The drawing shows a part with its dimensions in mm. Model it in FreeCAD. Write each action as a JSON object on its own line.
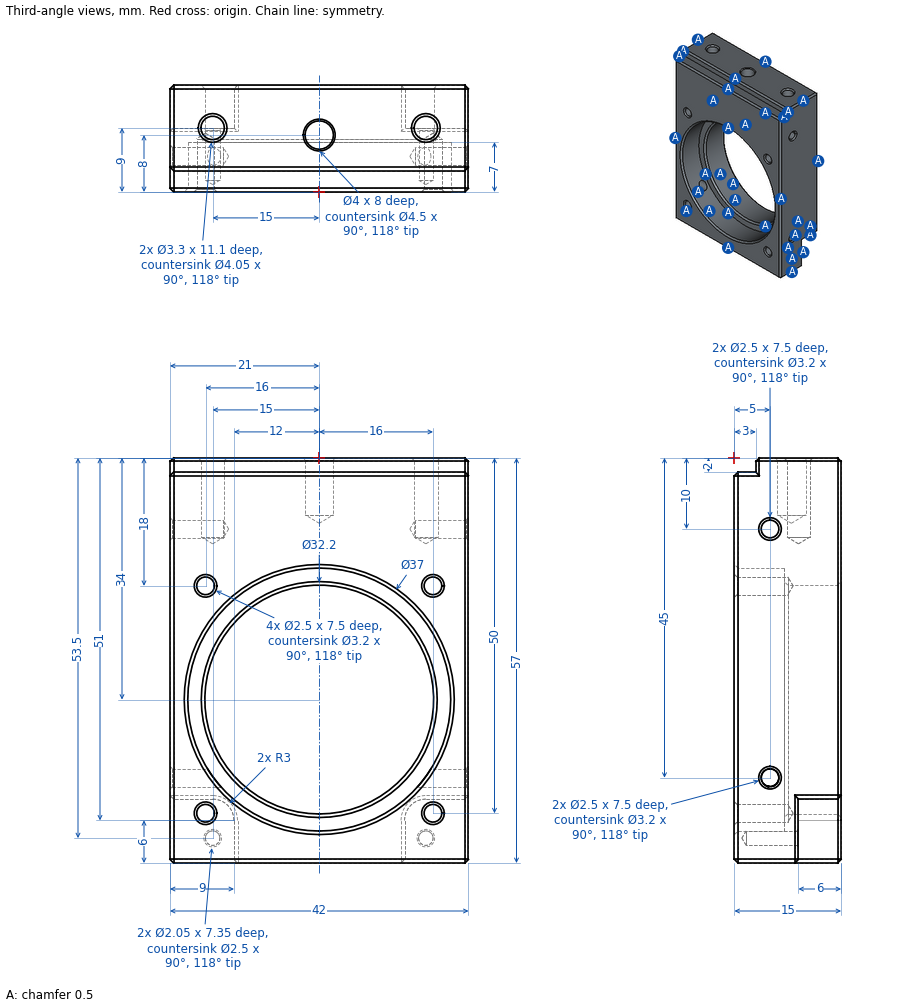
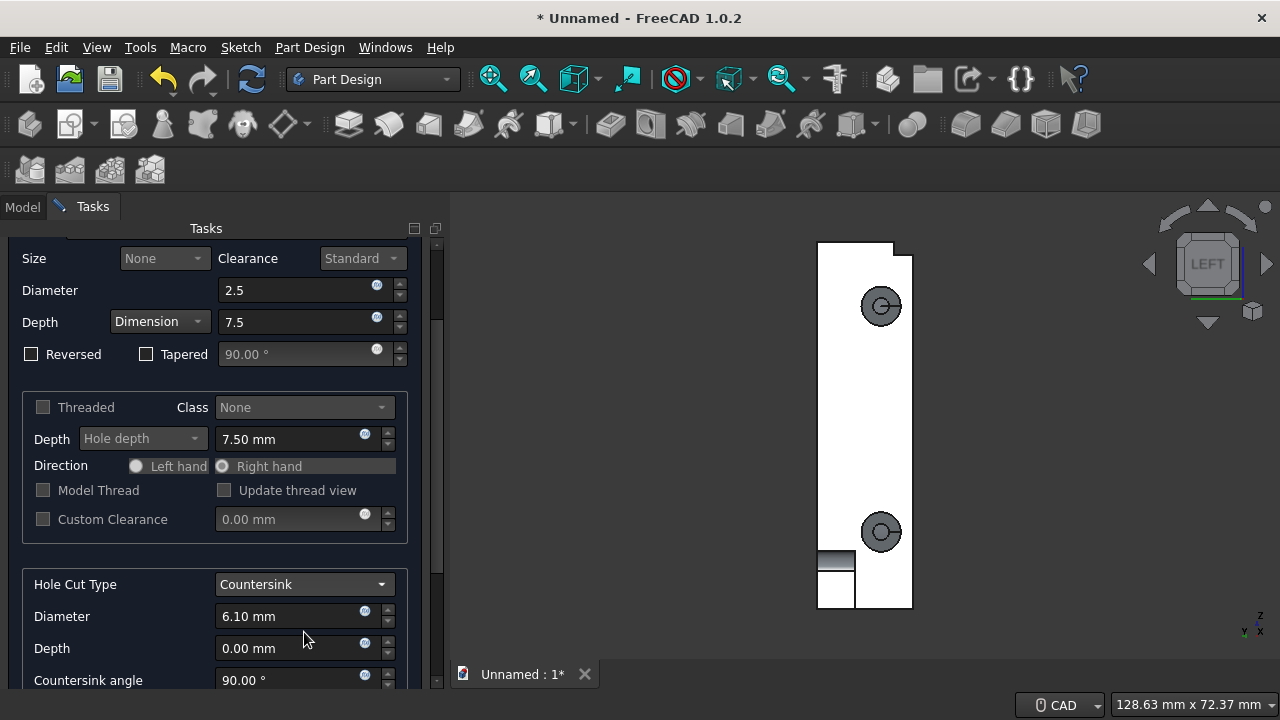
{"action": "triple_click", "coordinate": [298, 616]}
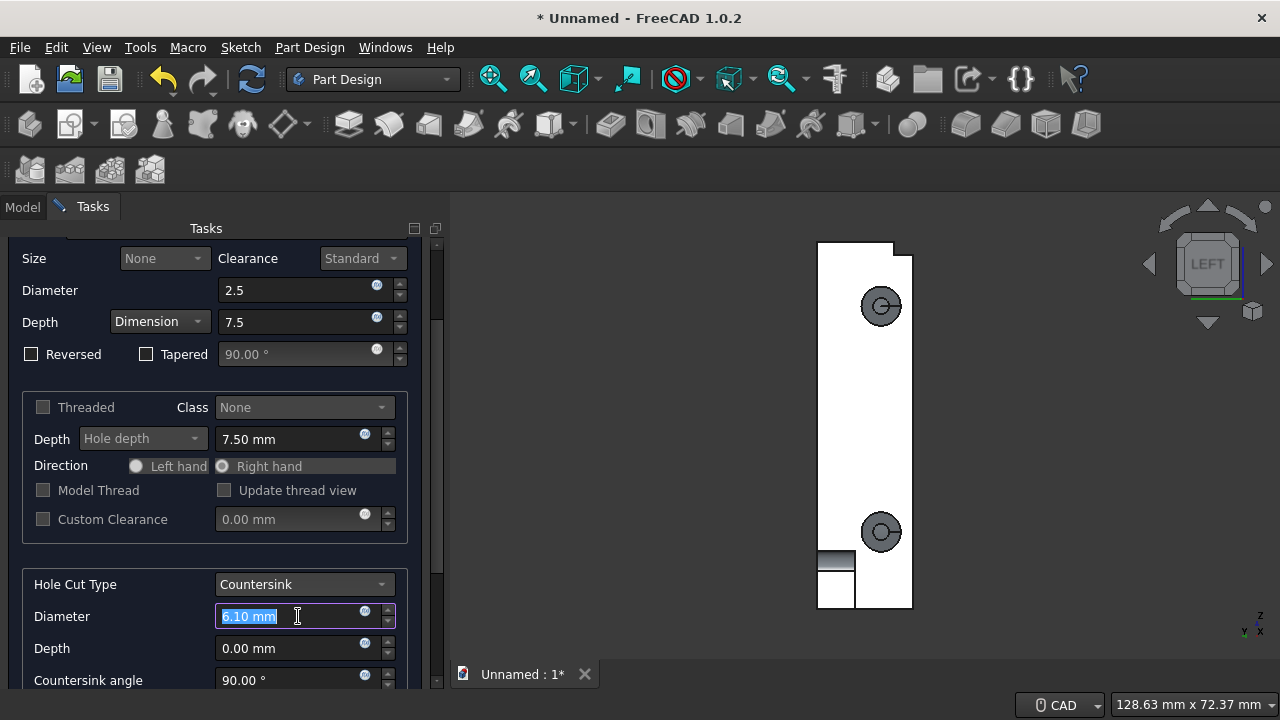
{"action": "type", "text": "3.2"}
{"action": "key", "text": "Tab"}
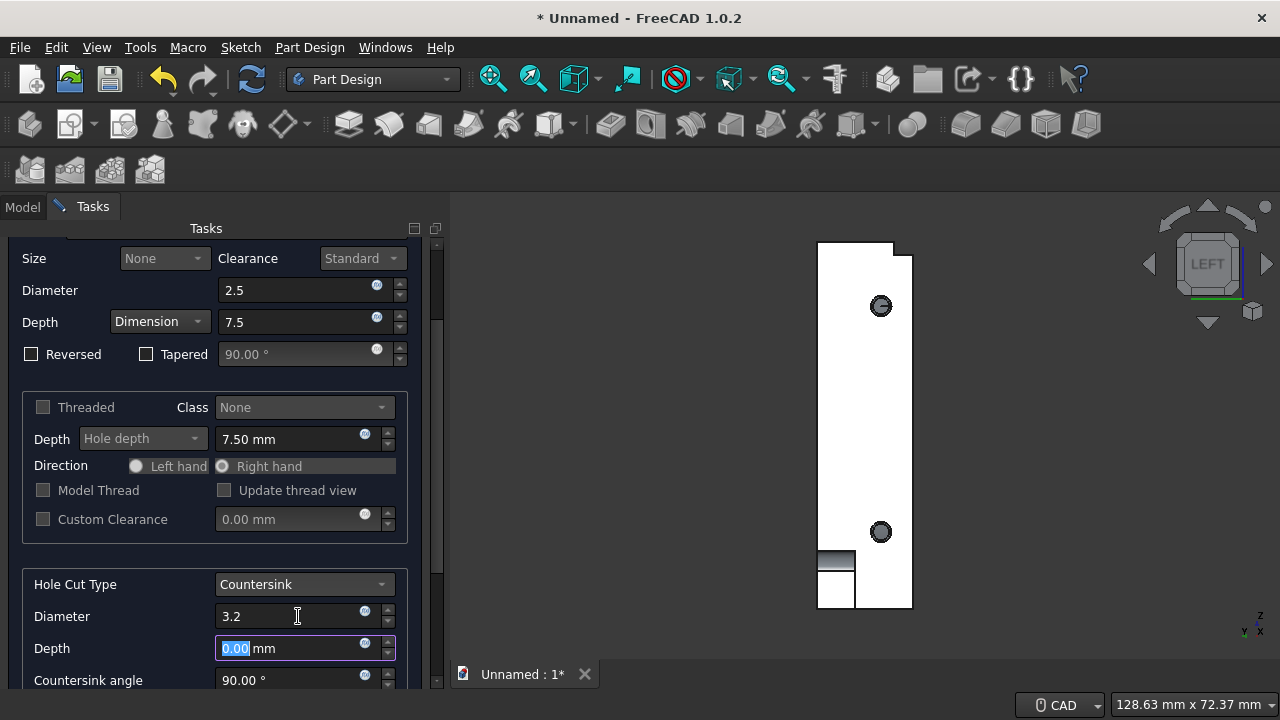
{"action": "scroll", "coordinate": [437, 463], "scroll_direction": "up", "scroll_amount": 3}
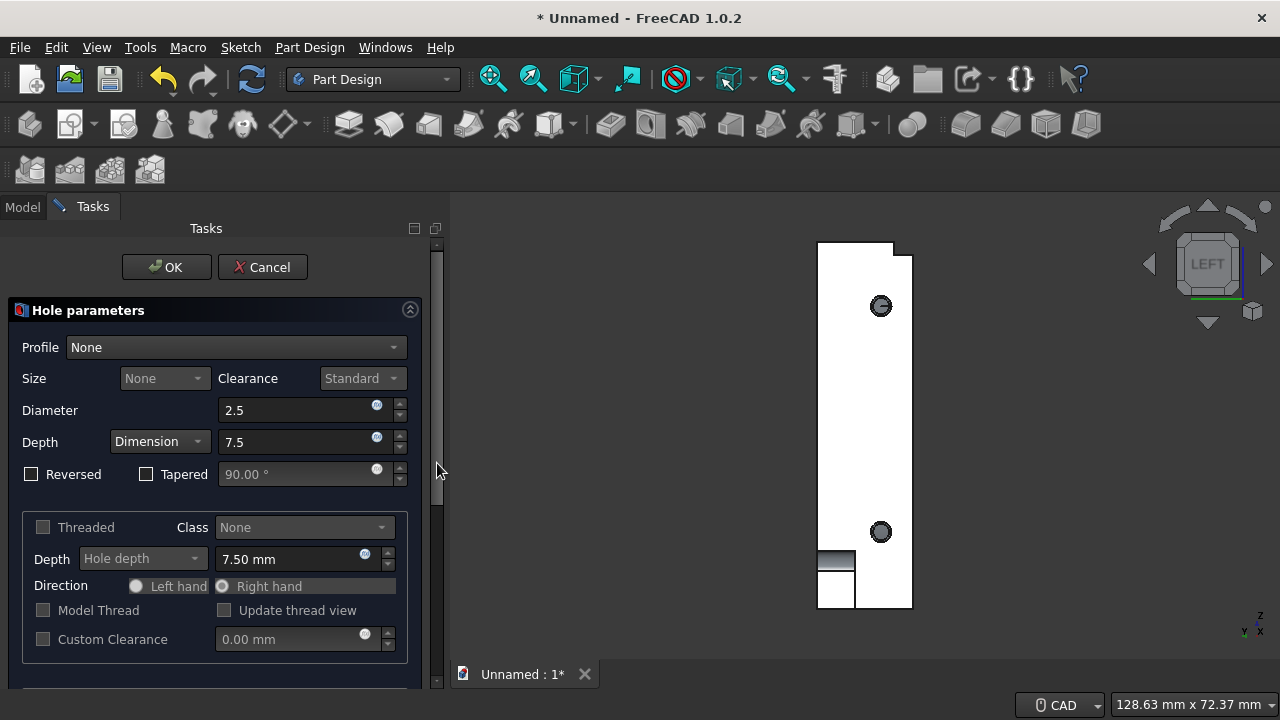
{"action": "left_click", "coordinate": [167, 267]}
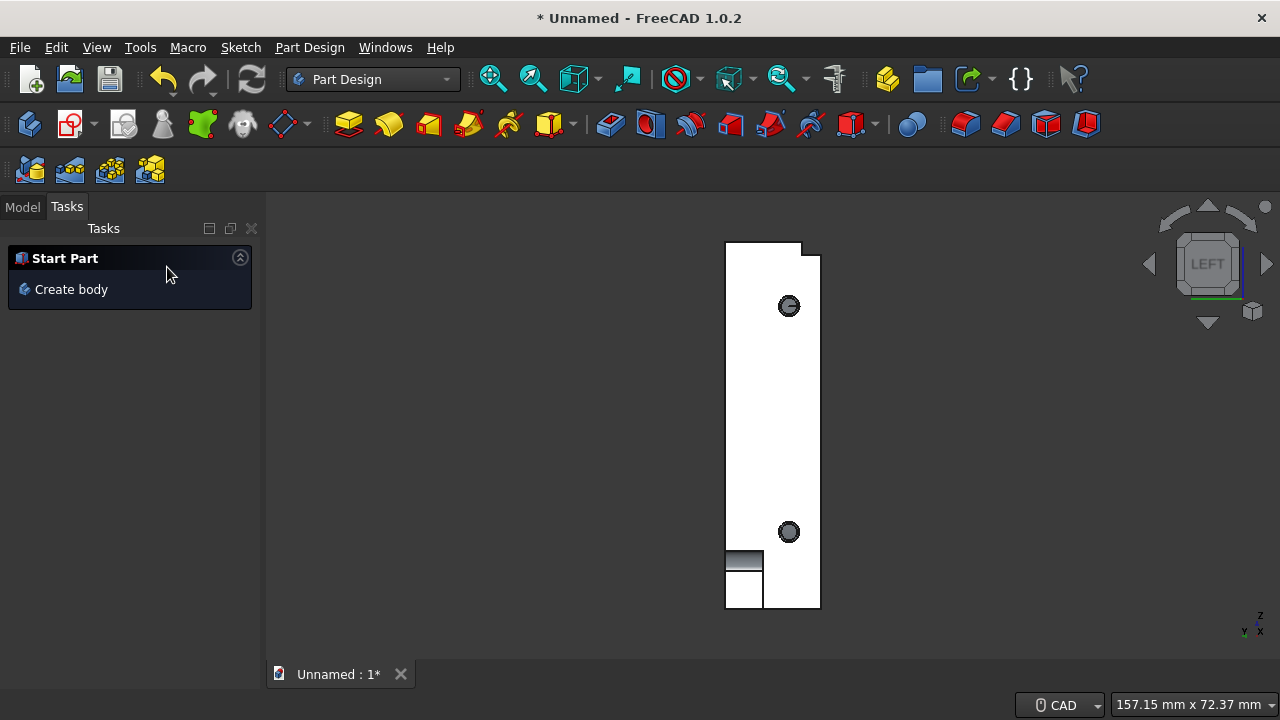
{"action": "key", "text": "0"}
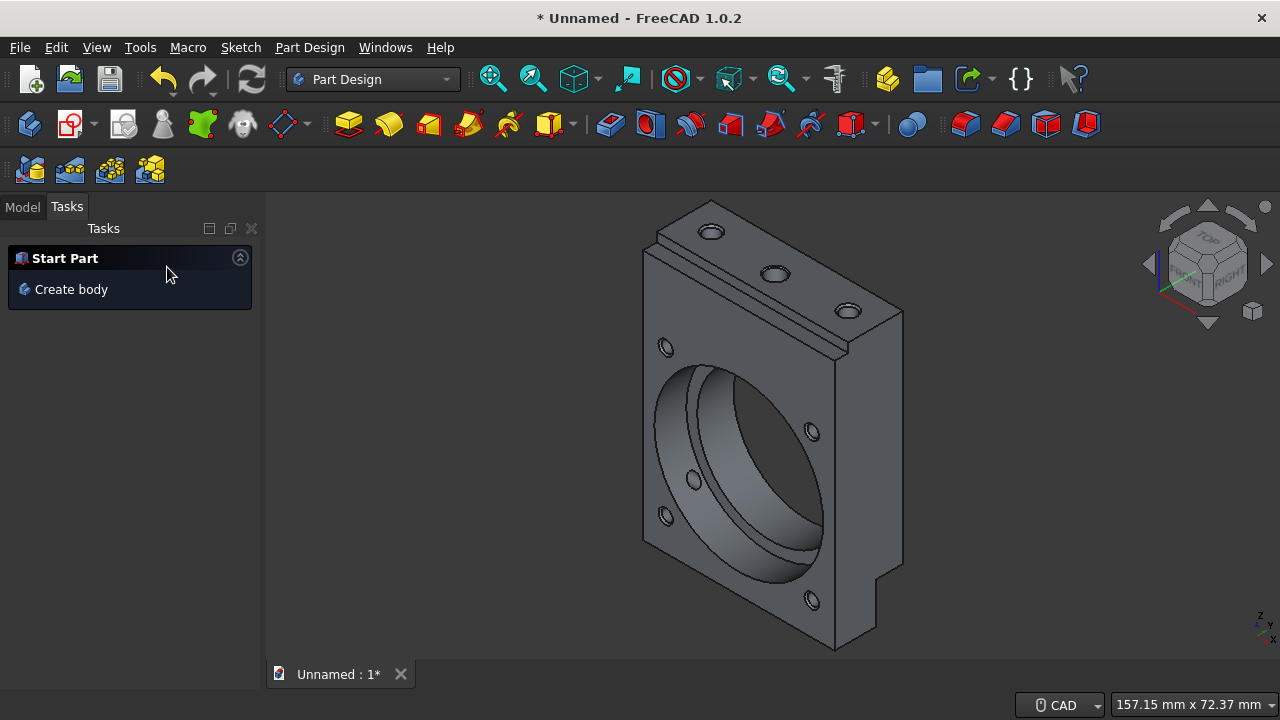
{"action": "left_click", "coordinate": [869, 394]}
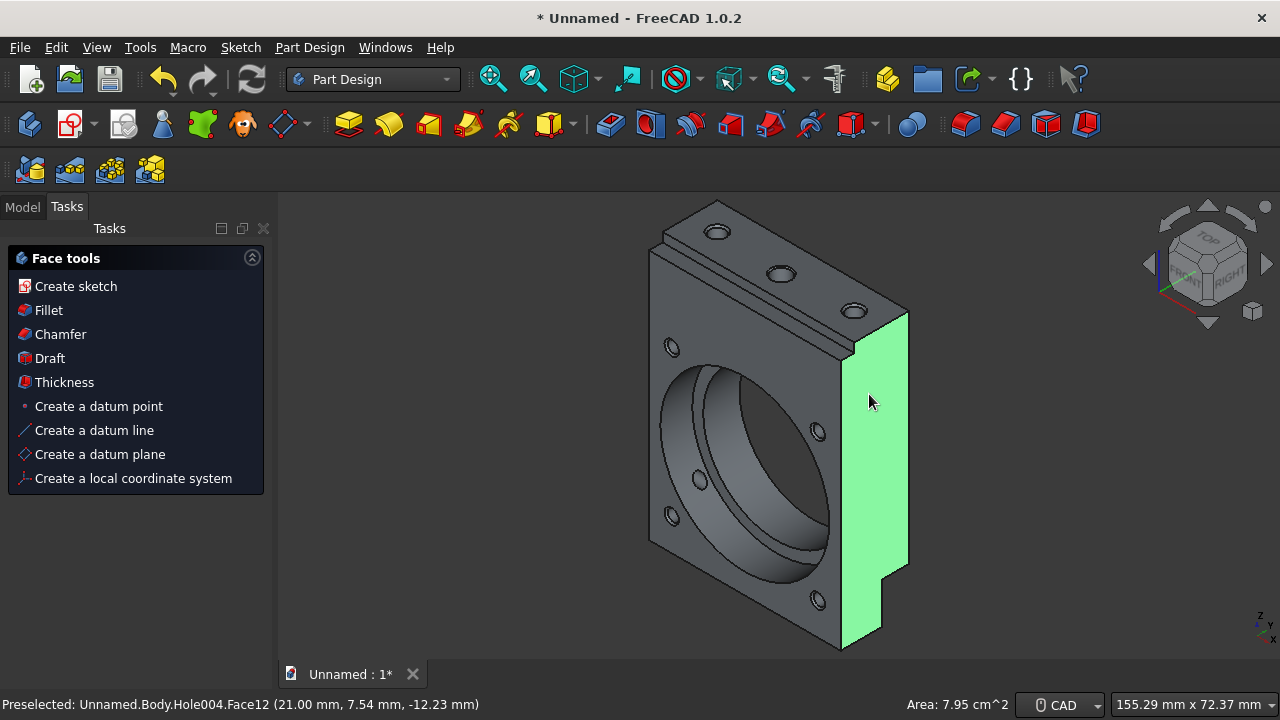
{"action": "left_click", "coordinate": [70, 124]}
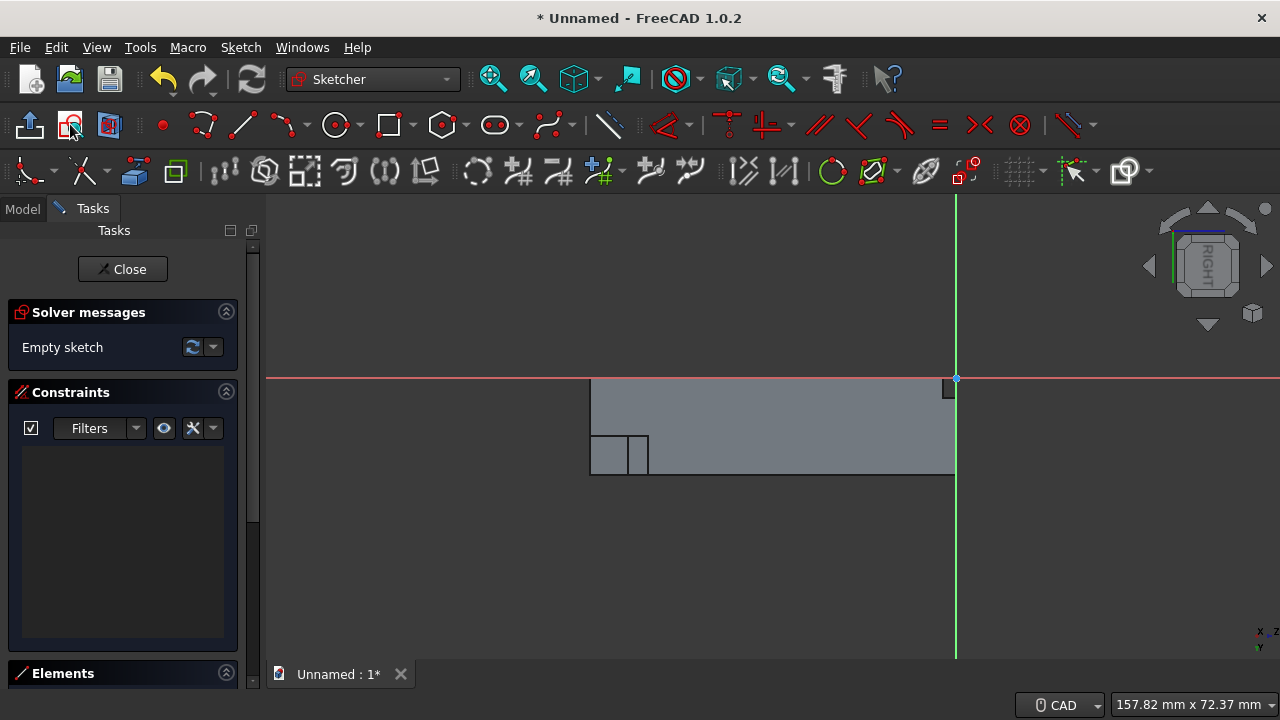
{"action": "scroll", "coordinate": [933, 364], "scroll_direction": "up", "scroll_amount": 3}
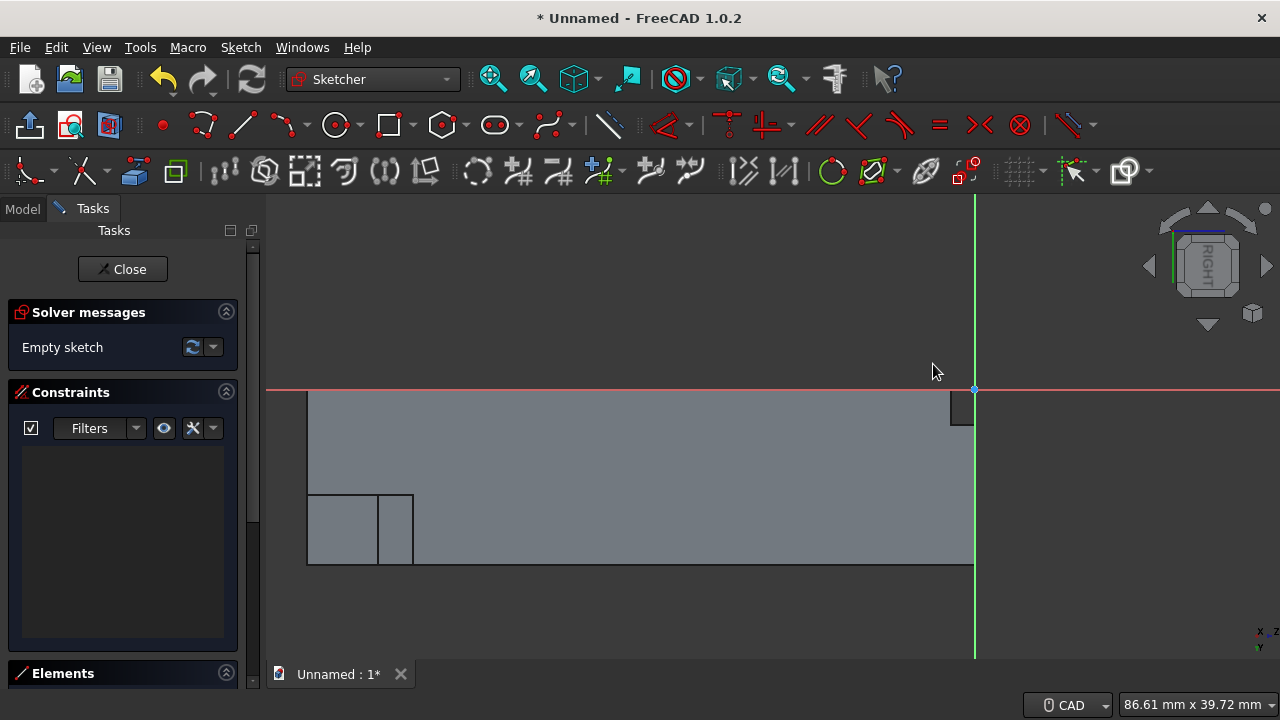
{"action": "key", "text": "g c"}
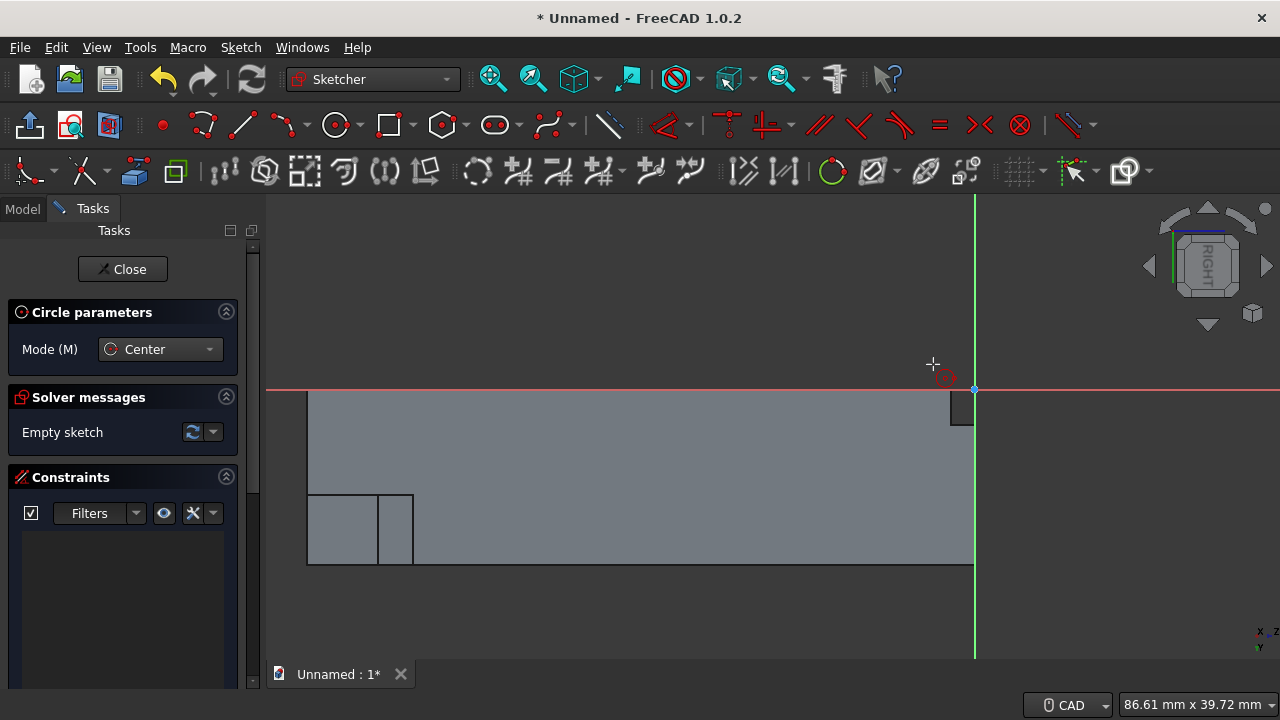
{"action": "scroll", "coordinate": [857, 448], "scroll_direction": "up", "scroll_amount": 3}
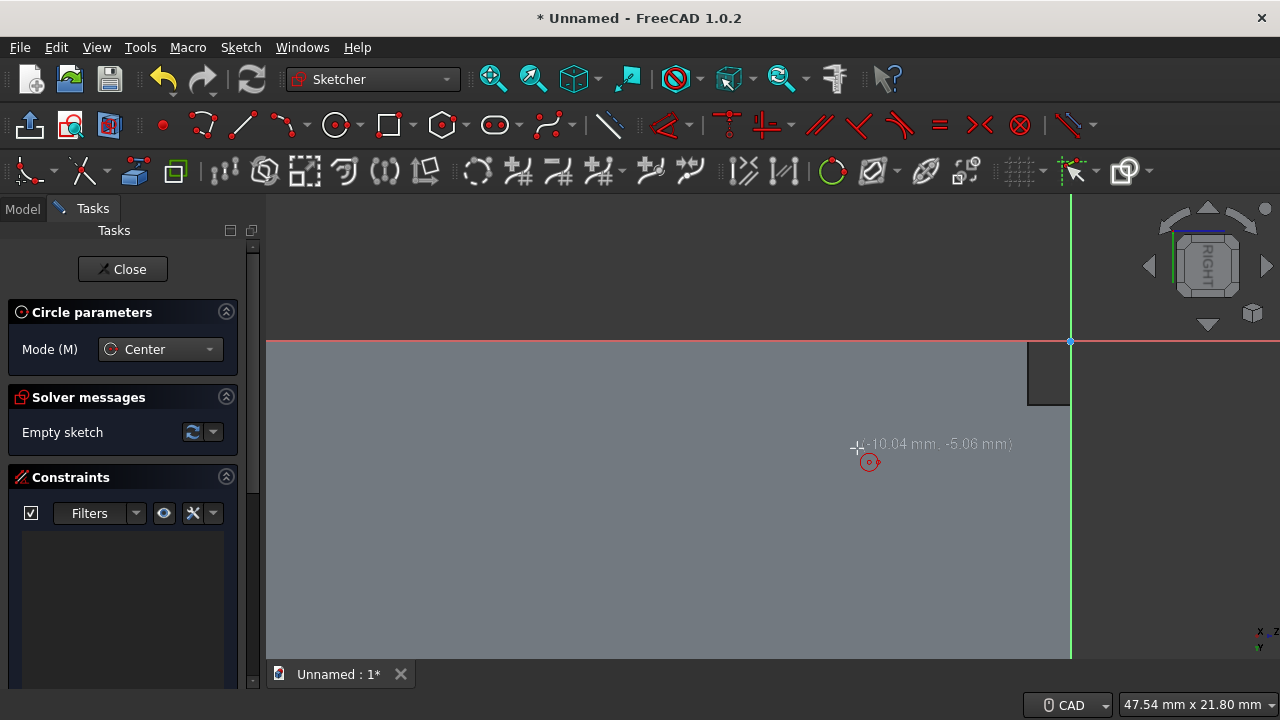
{"action": "left_click", "coordinate": [857, 448]}
{"action": "mouse_move", "coordinate": [876, 429]}